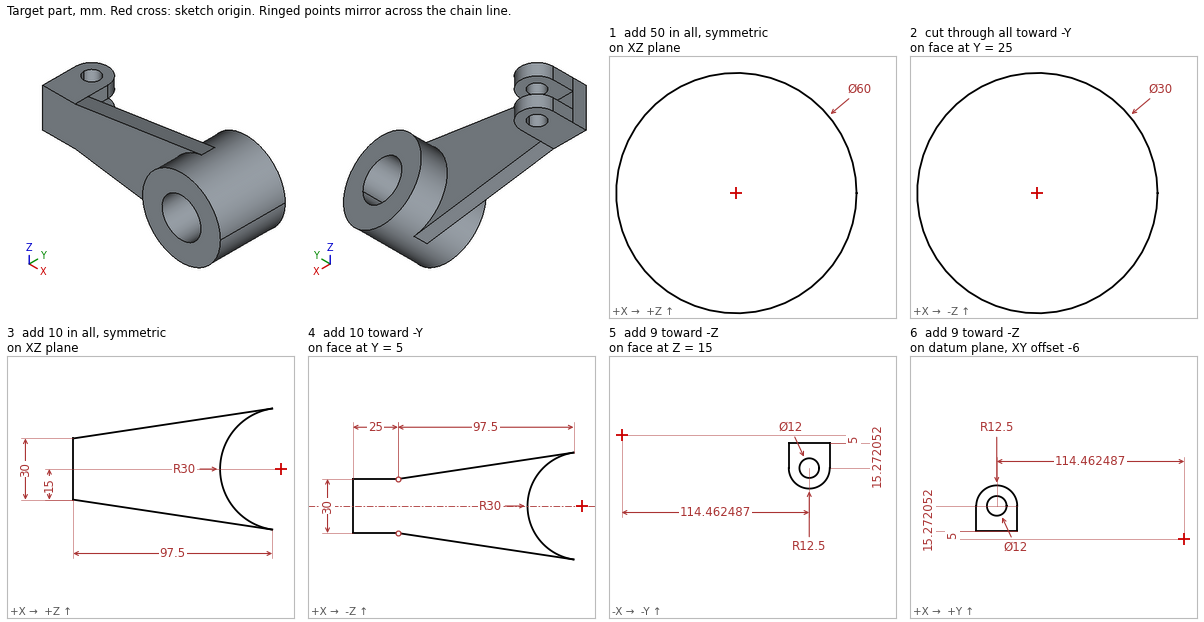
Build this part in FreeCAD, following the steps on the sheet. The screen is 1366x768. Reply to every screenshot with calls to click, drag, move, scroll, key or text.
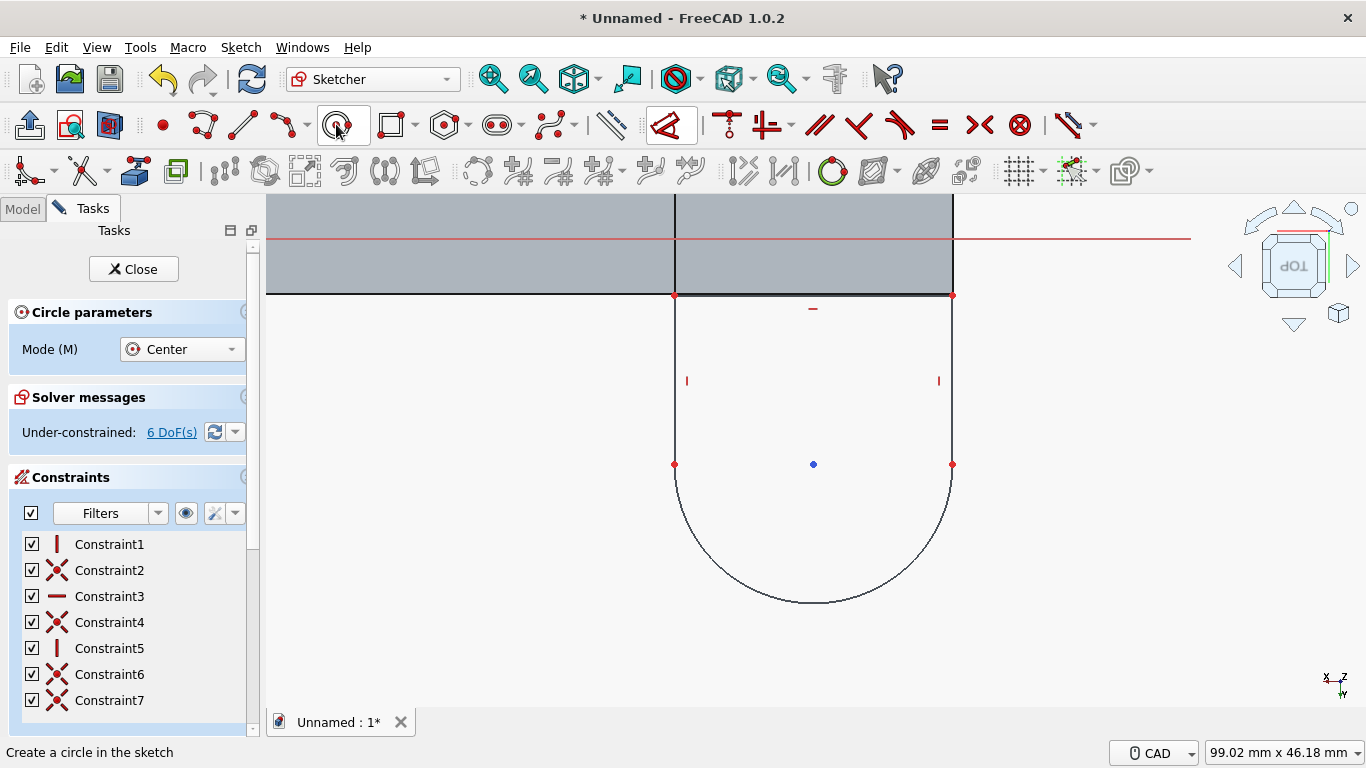
click(814, 464)
move(861, 417)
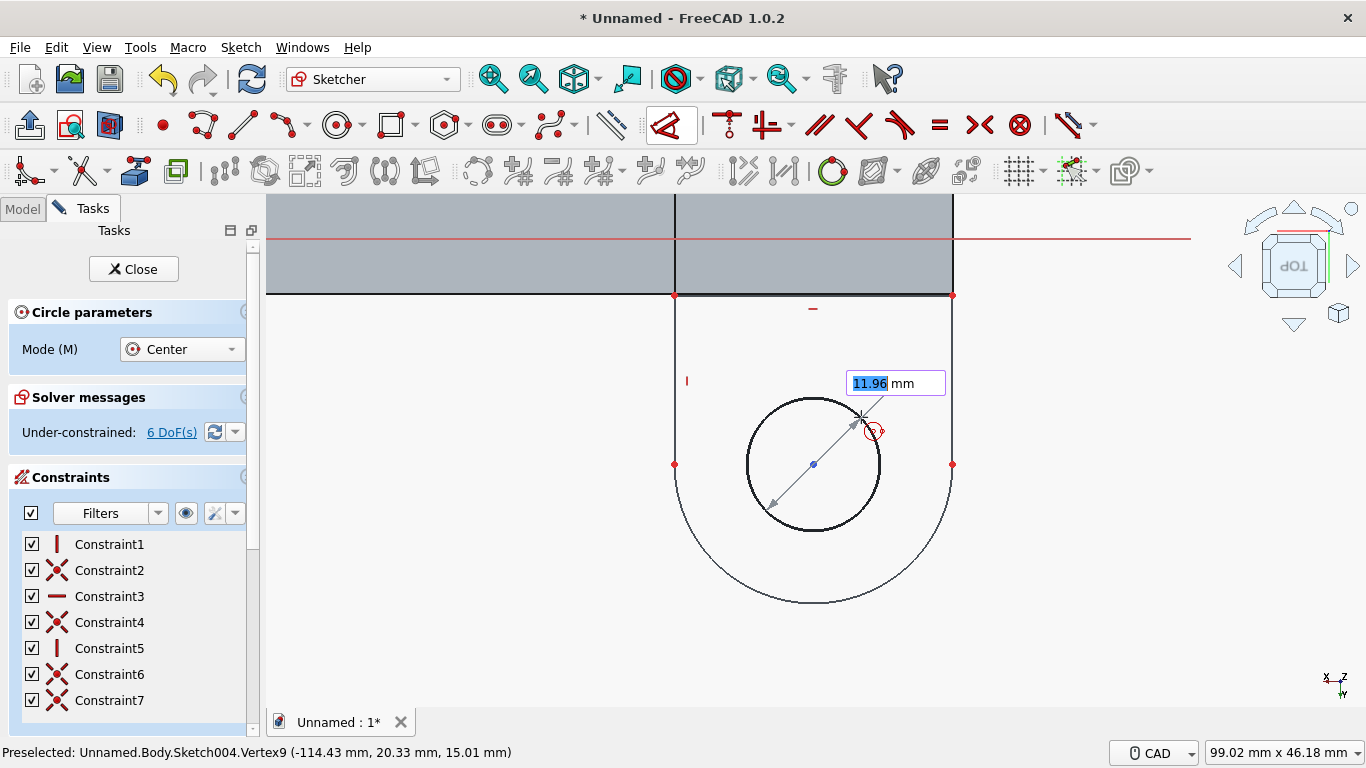
text(12)
key(Return)
key(Escape)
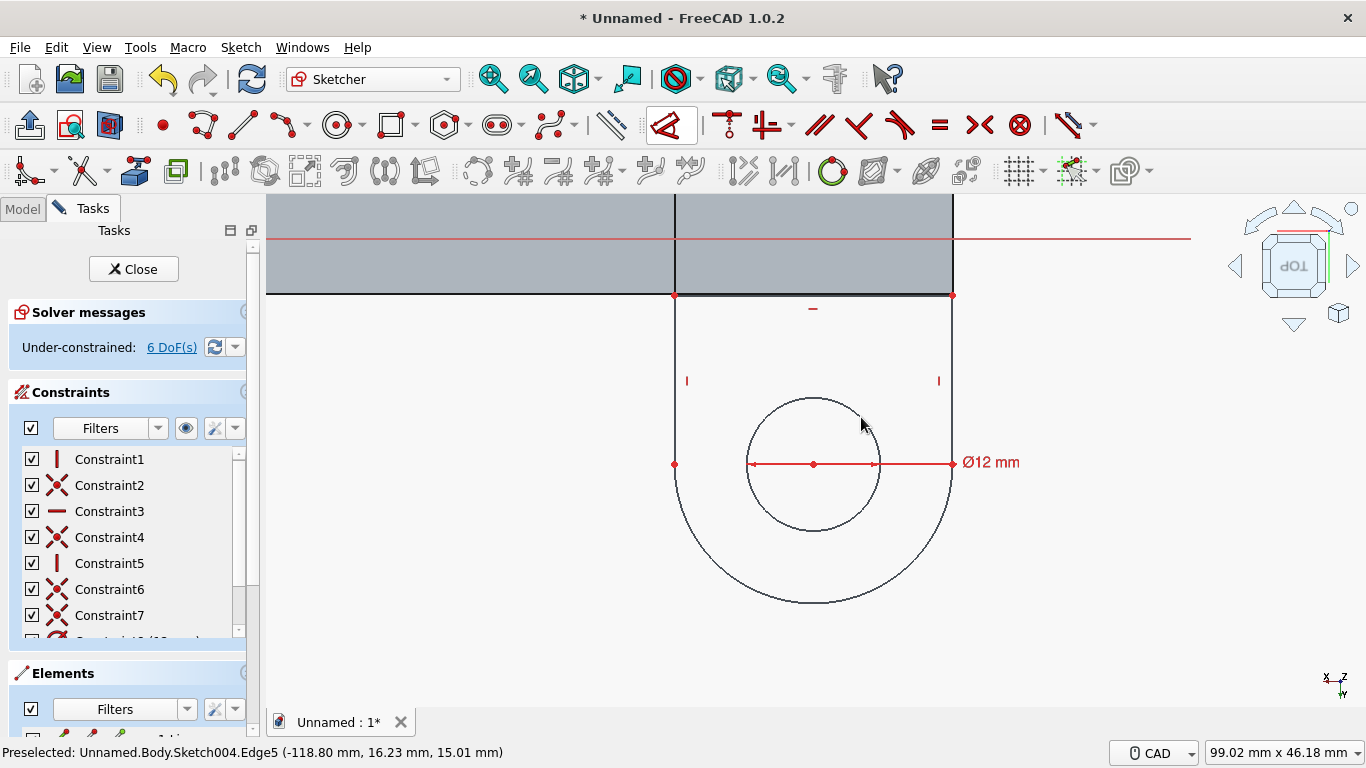
click(952, 414)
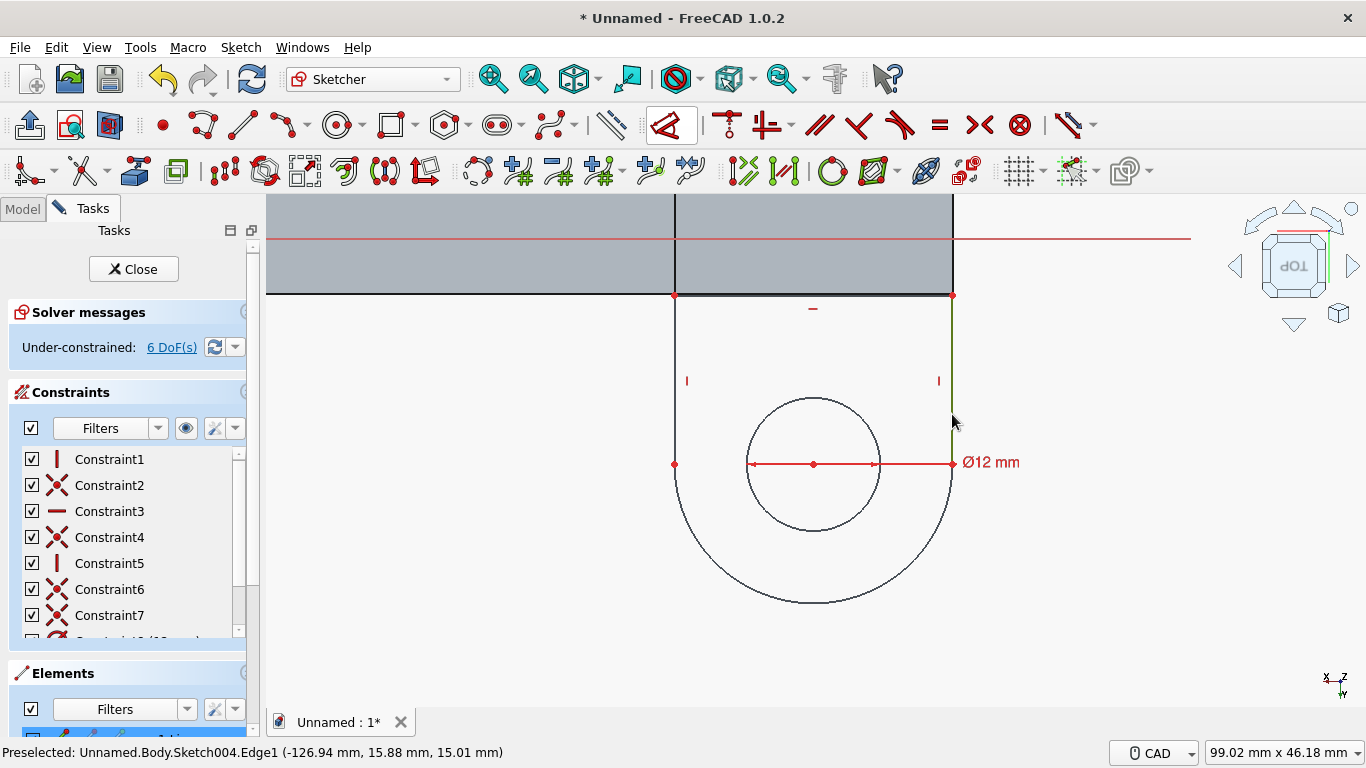
click(732, 577)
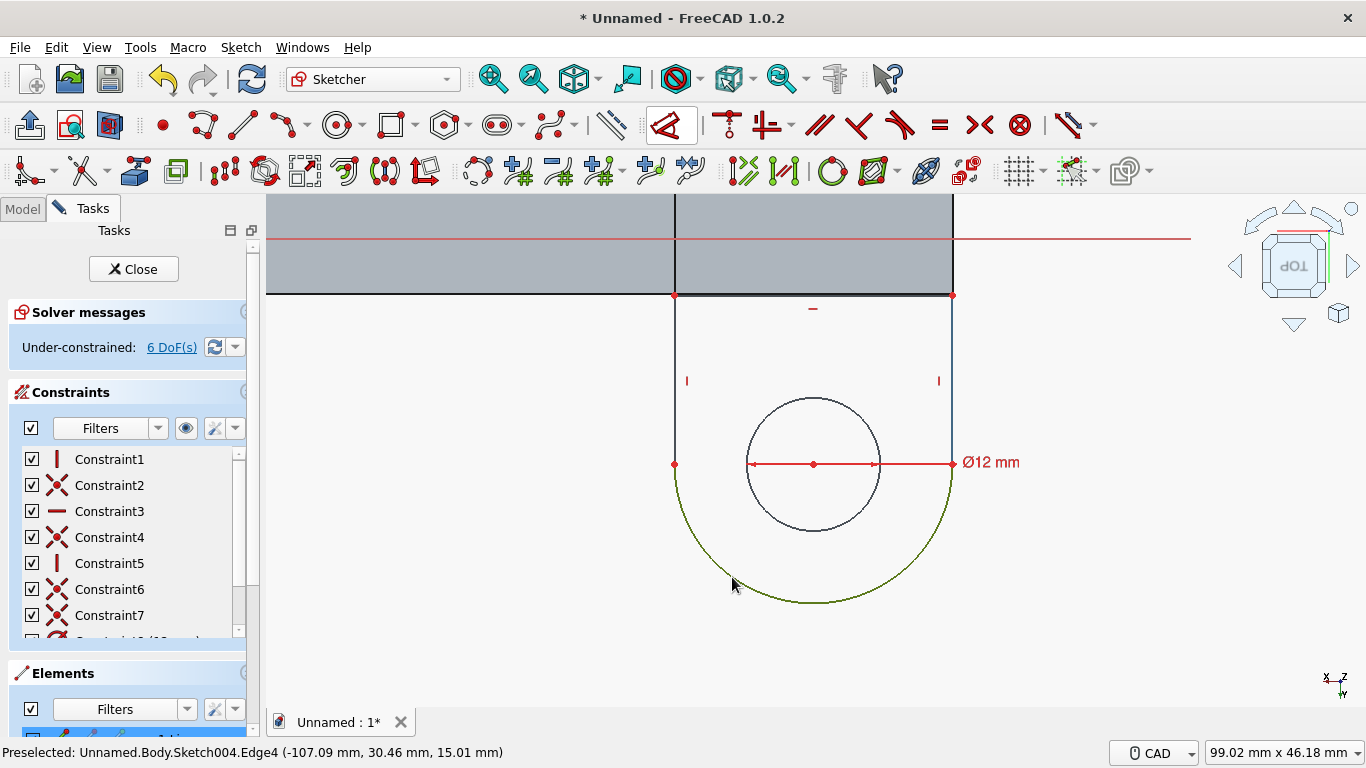
click(900, 126)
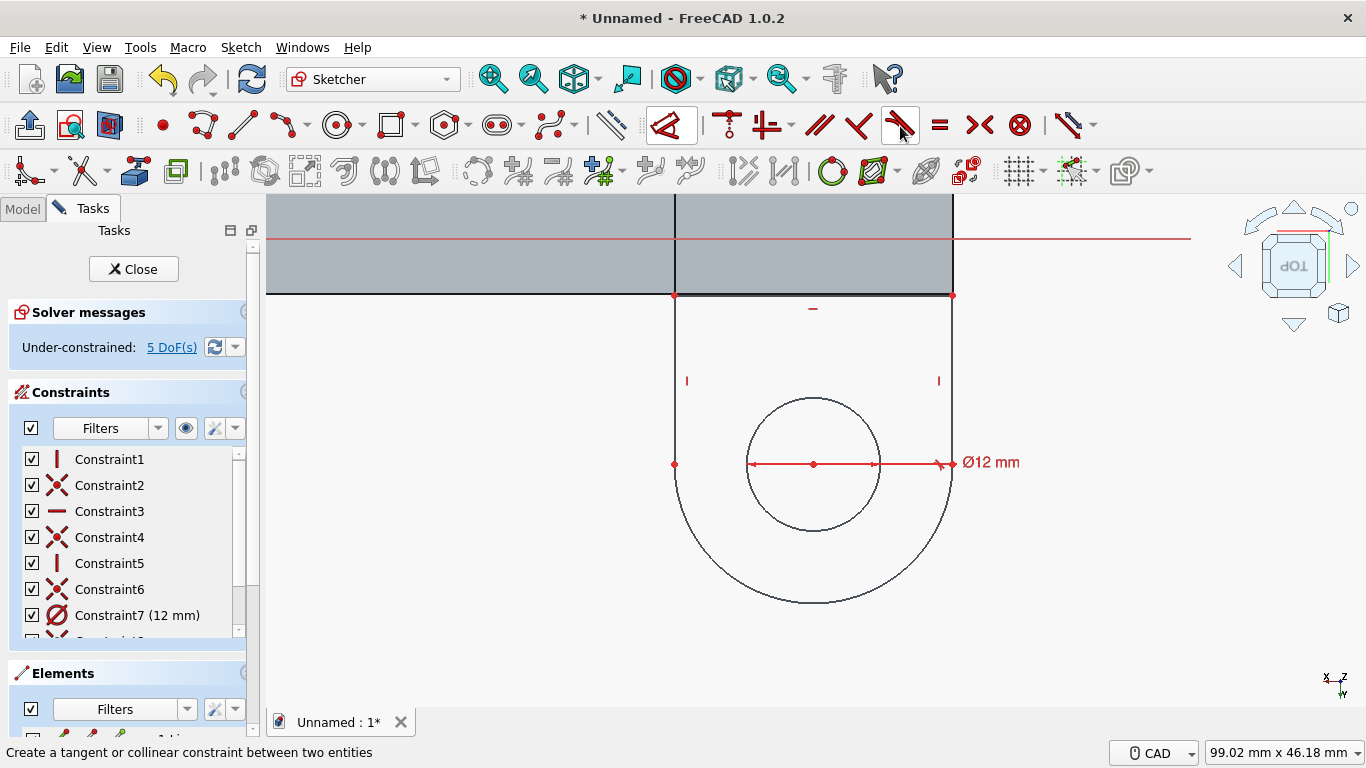
click(675, 346)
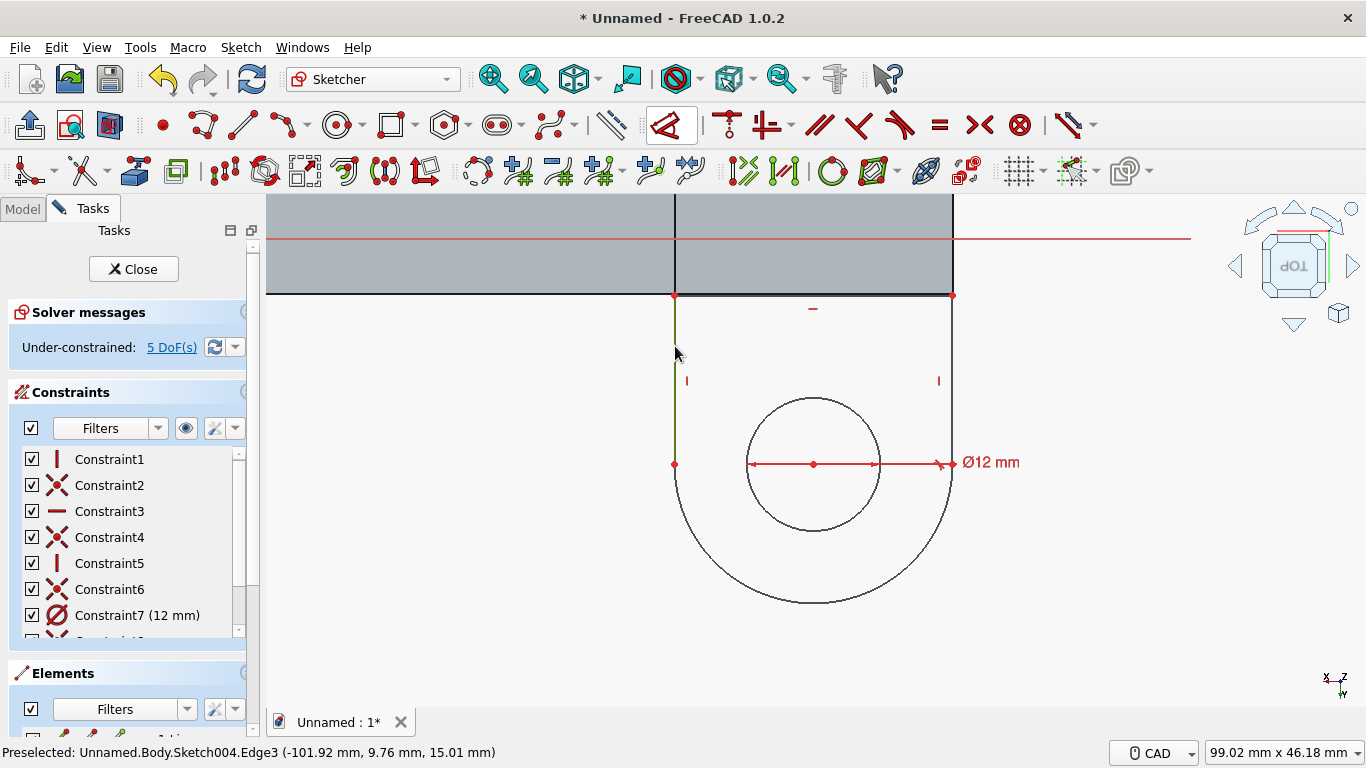
click(732, 577)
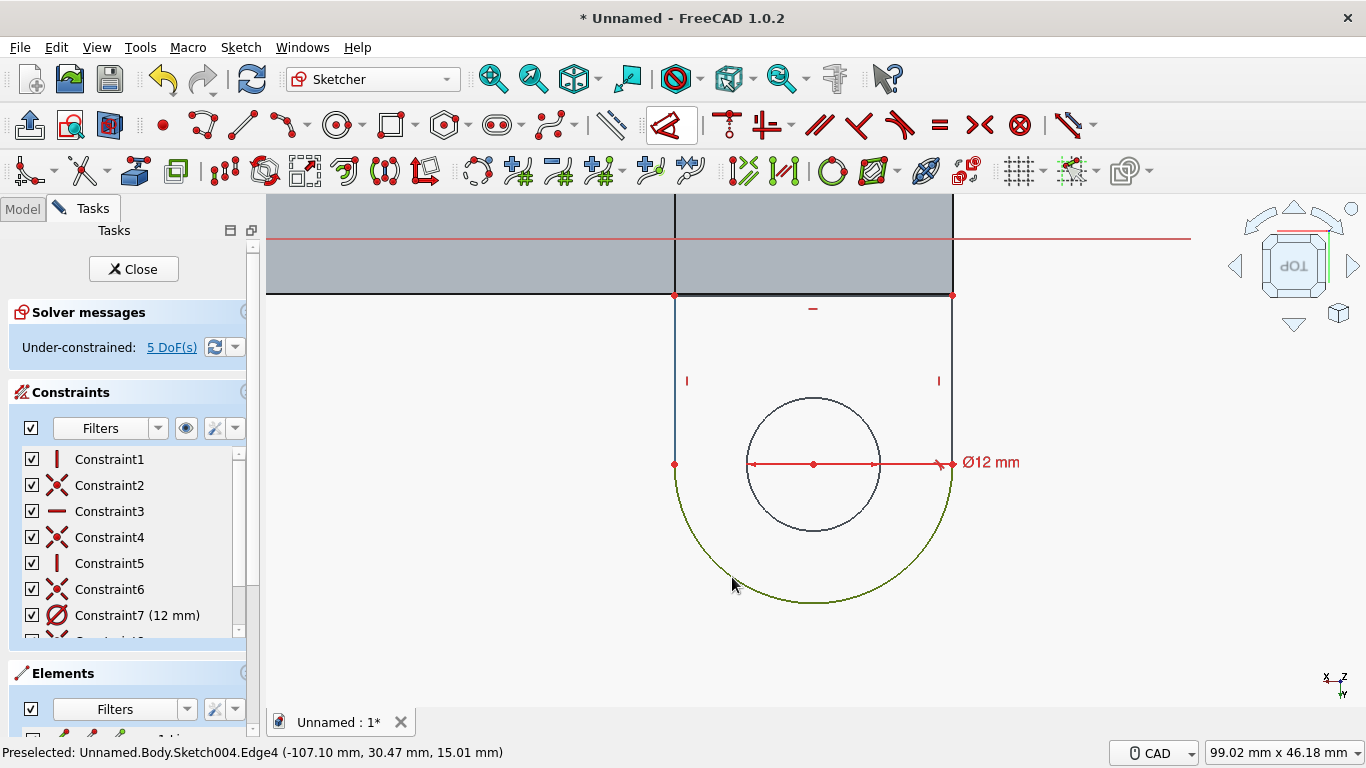
click(900, 126)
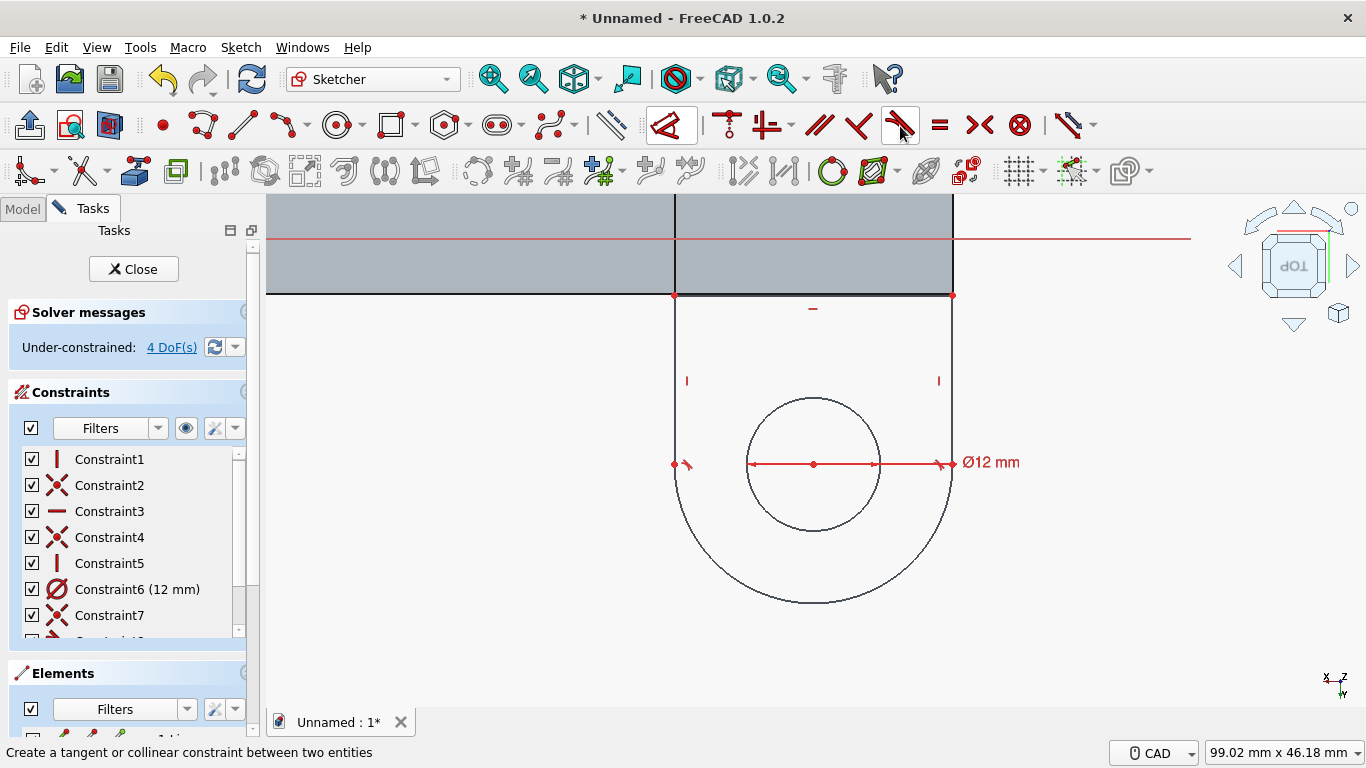
click(732, 577)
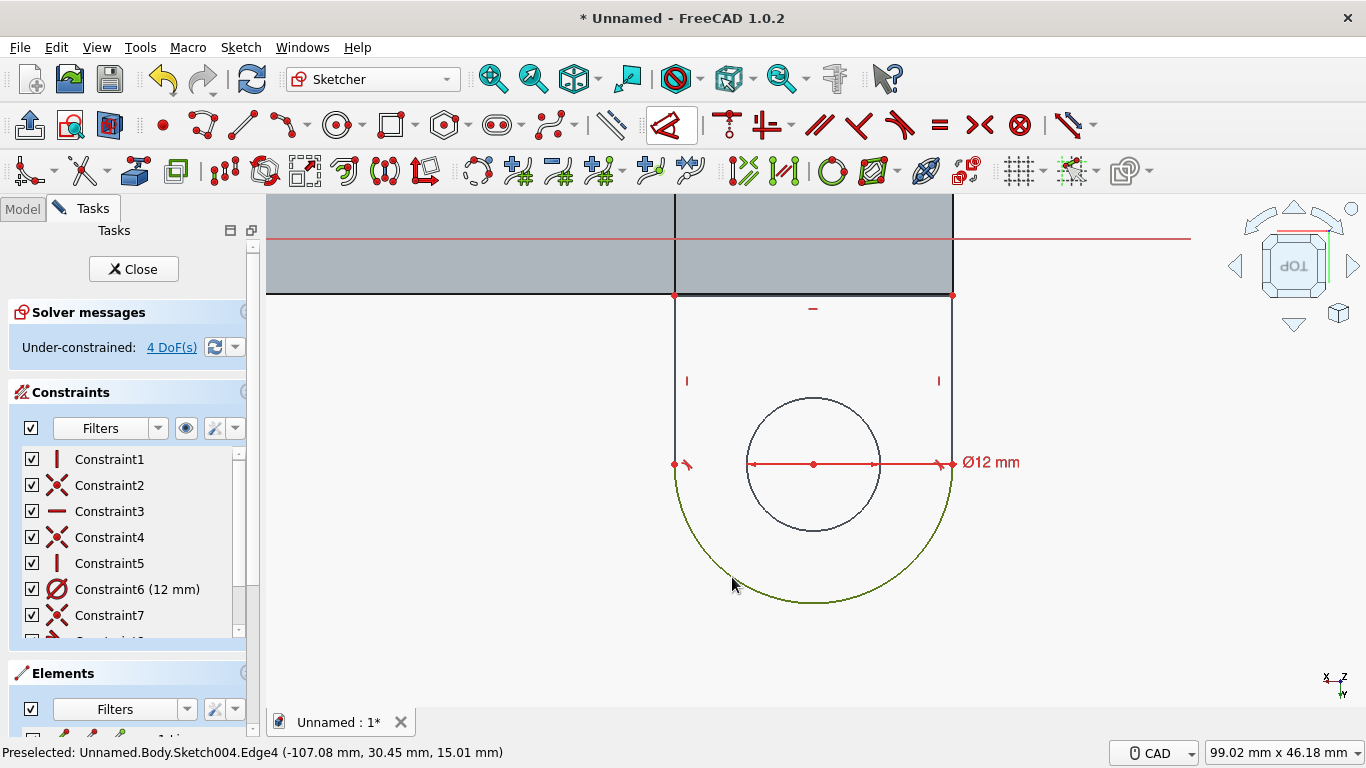
click(692, 126)